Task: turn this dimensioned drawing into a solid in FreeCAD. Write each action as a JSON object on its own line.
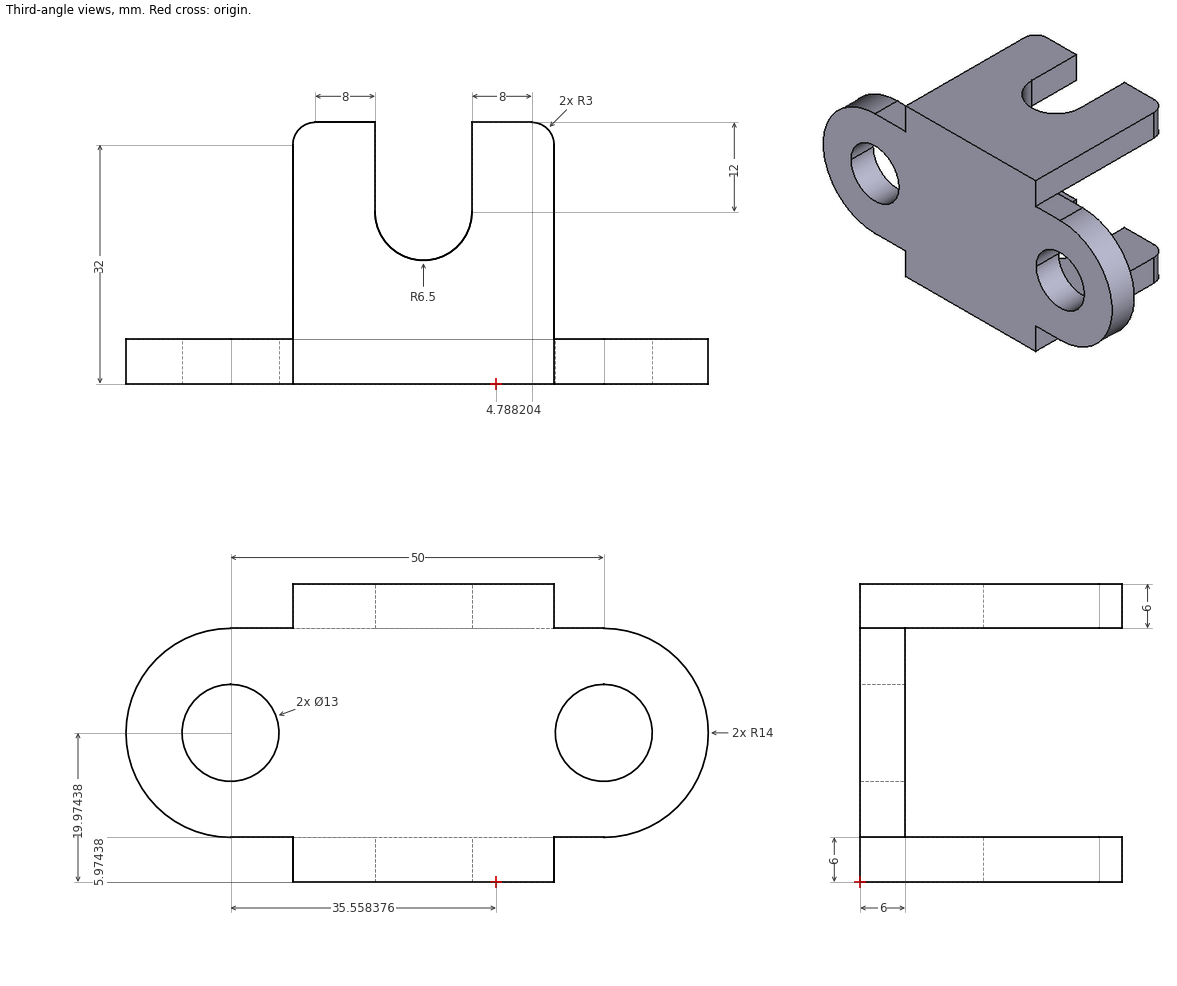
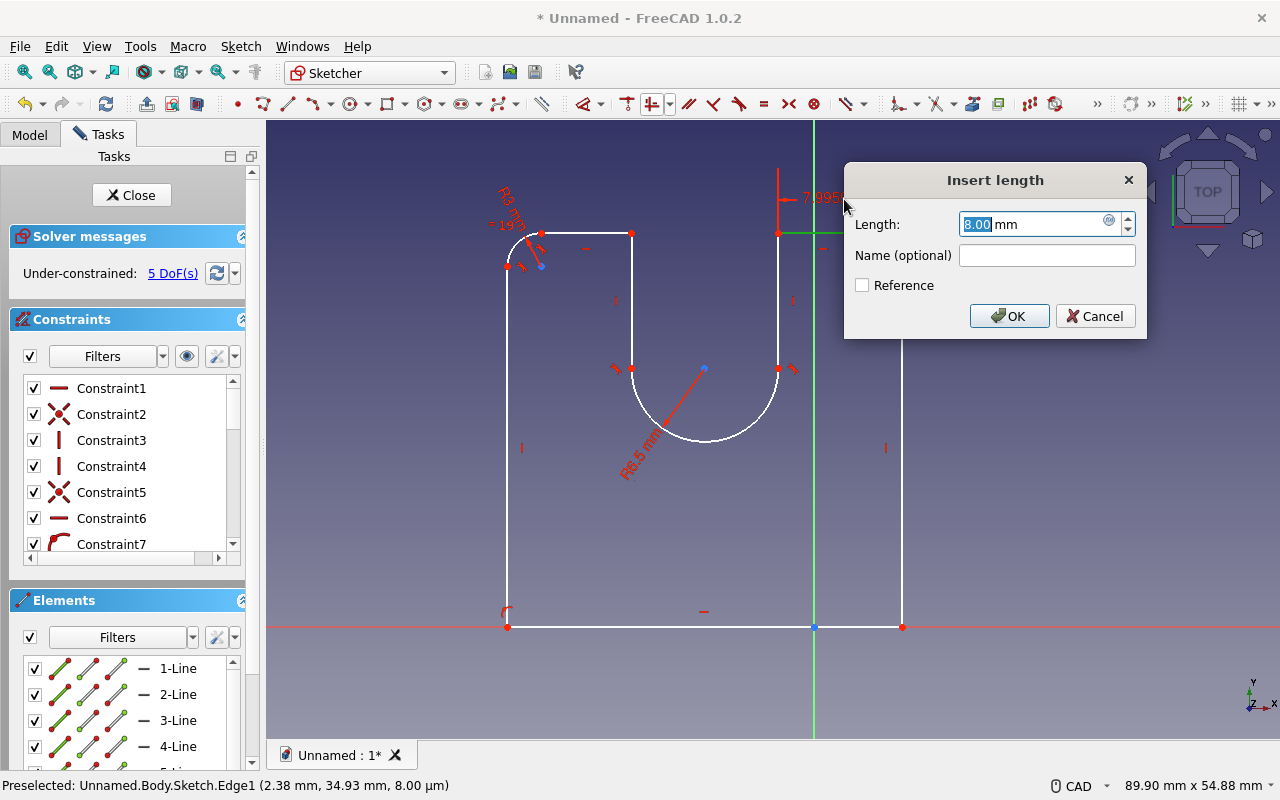
{"action": "type", "text": "8"}
{"action": "key", "text": "Return"}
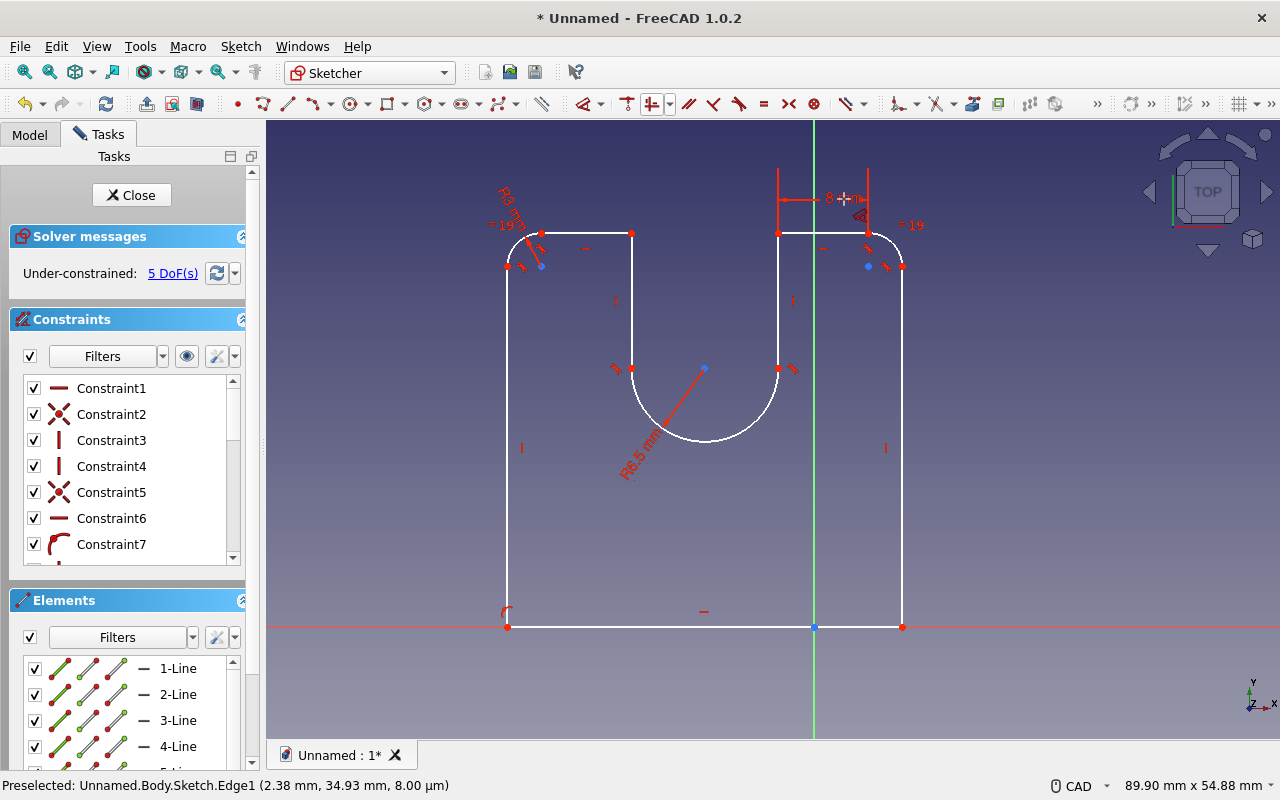
{"action": "left_click", "coordinate": [604, 233]}
{"action": "left_click", "coordinate": [586, 199]}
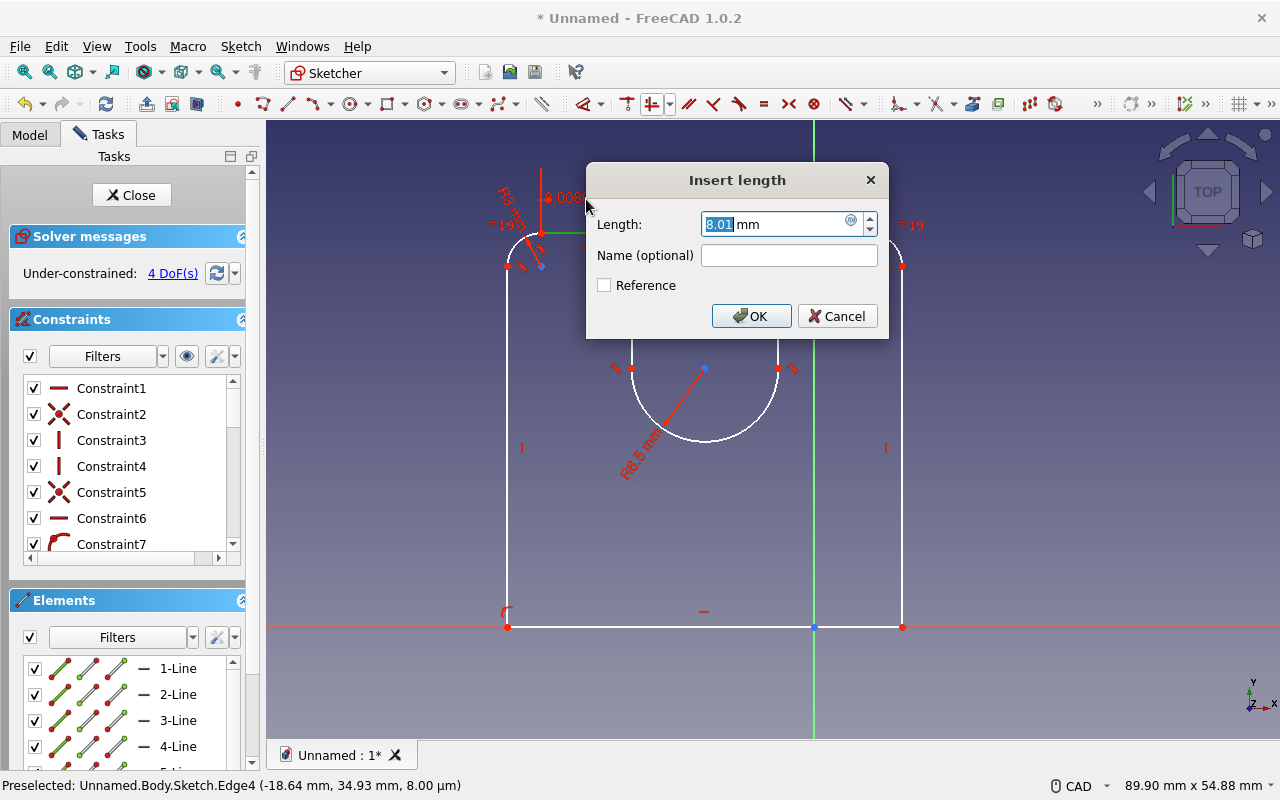
{"action": "type", "text": "8"}
{"action": "key", "text": "Return"}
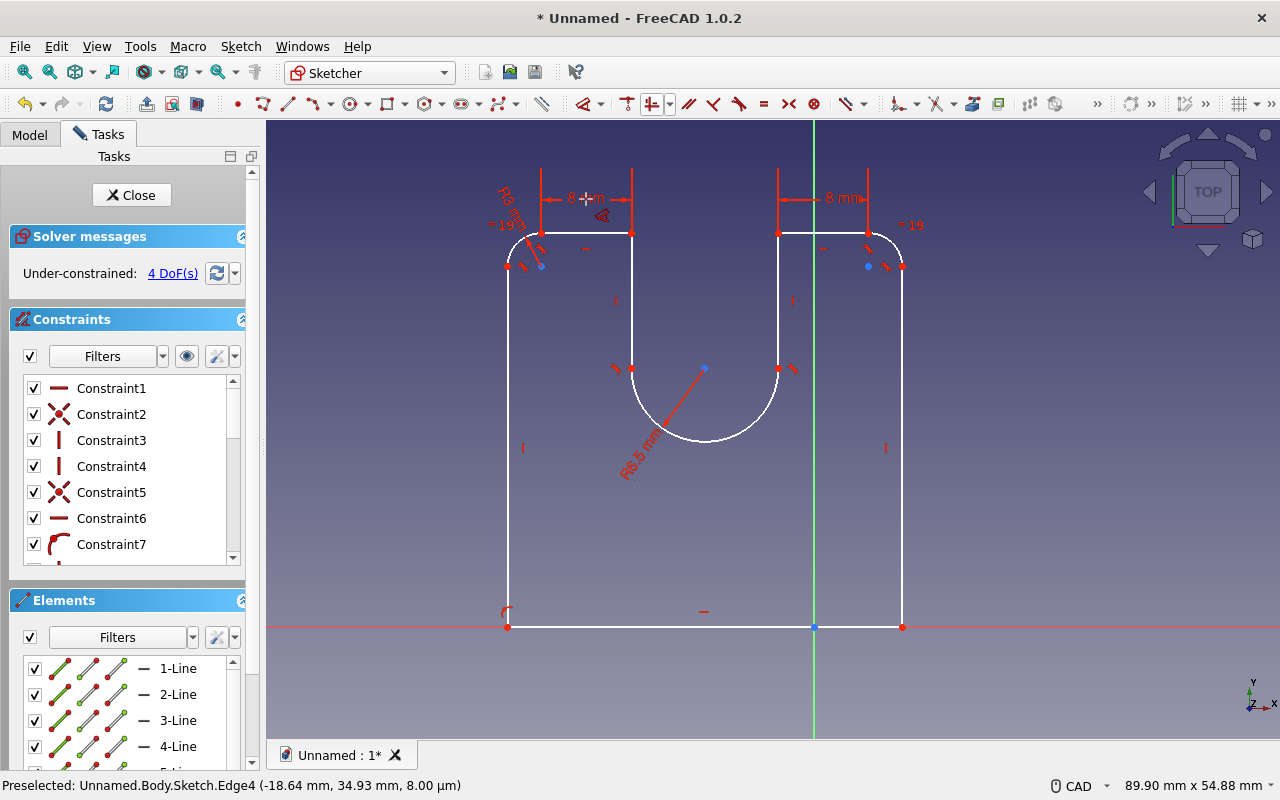
{"action": "left_click", "coordinate": [778, 274]}
{"action": "left_click", "coordinate": [744, 301]}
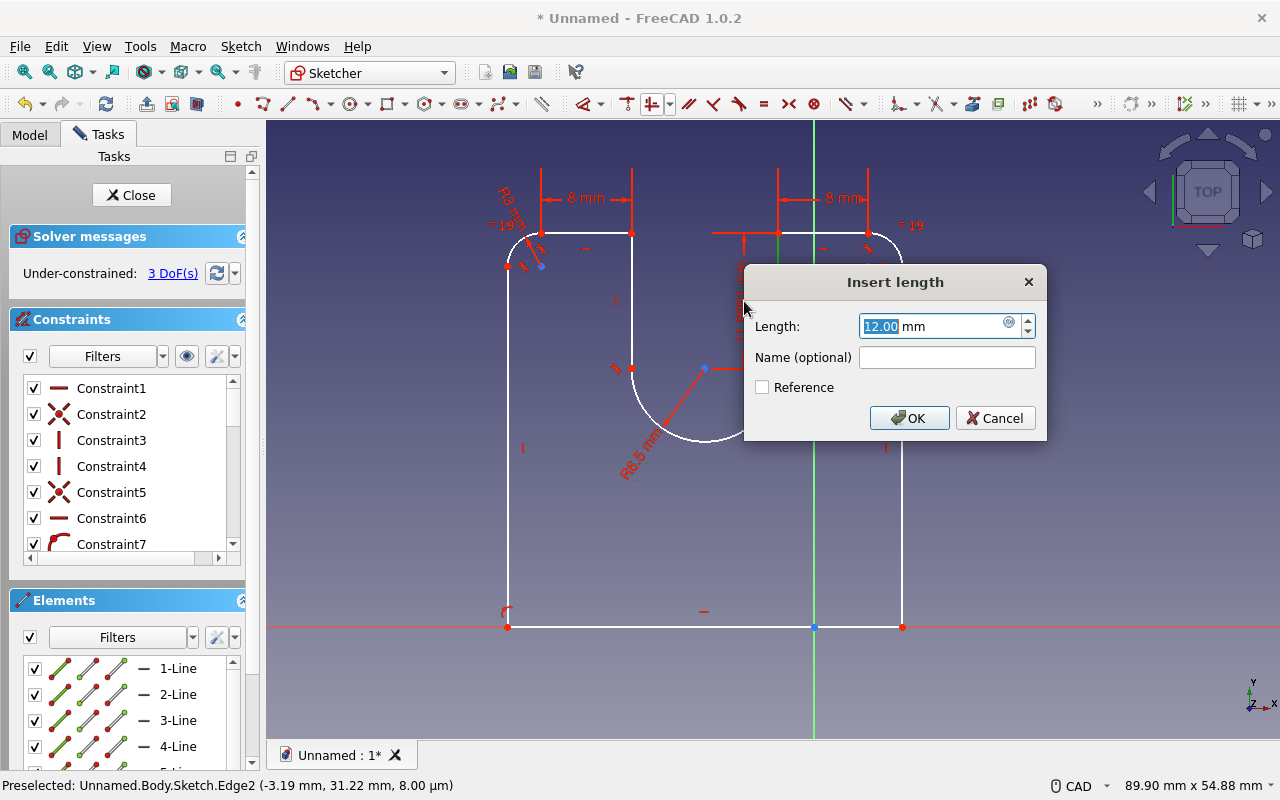
{"action": "type", "text": "12"}
{"action": "key", "text": "Return"}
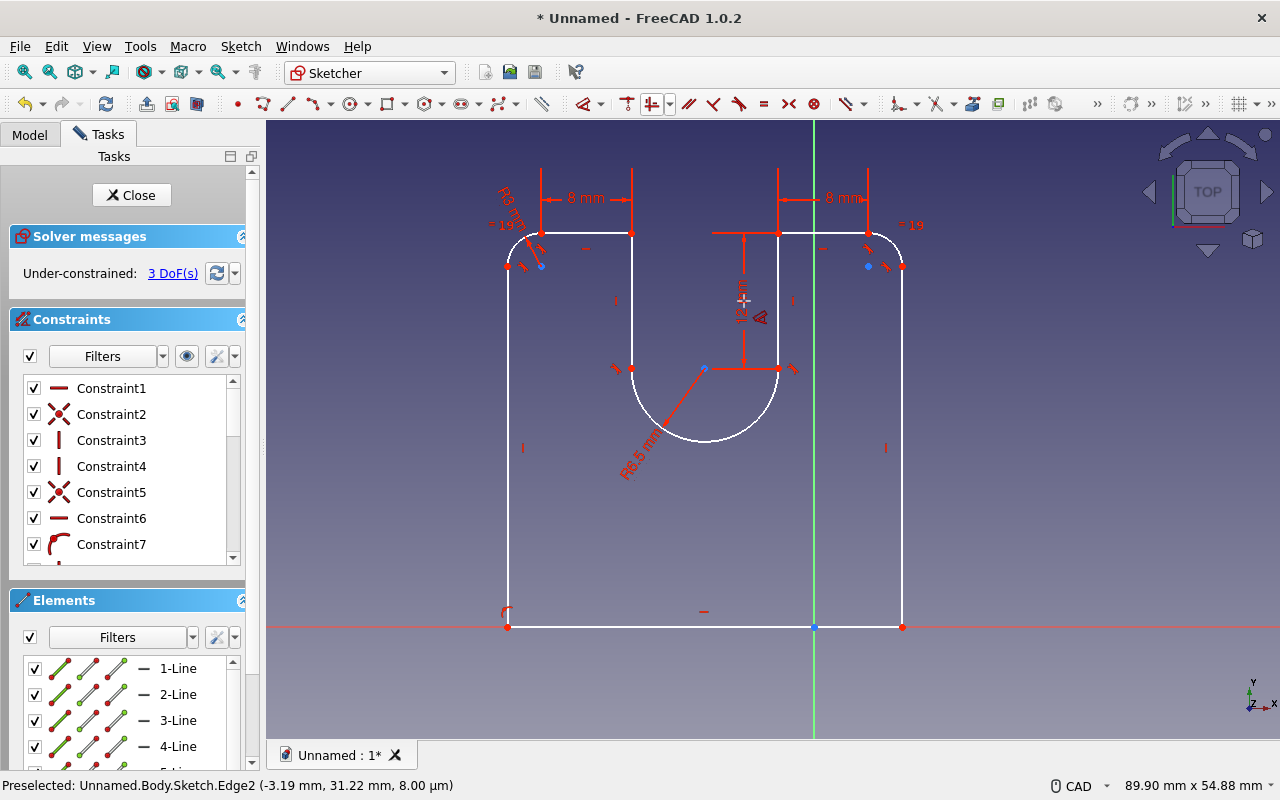
{"action": "left_click", "coordinate": [632, 328]}
{"action": "left_click", "coordinate": [598, 301]}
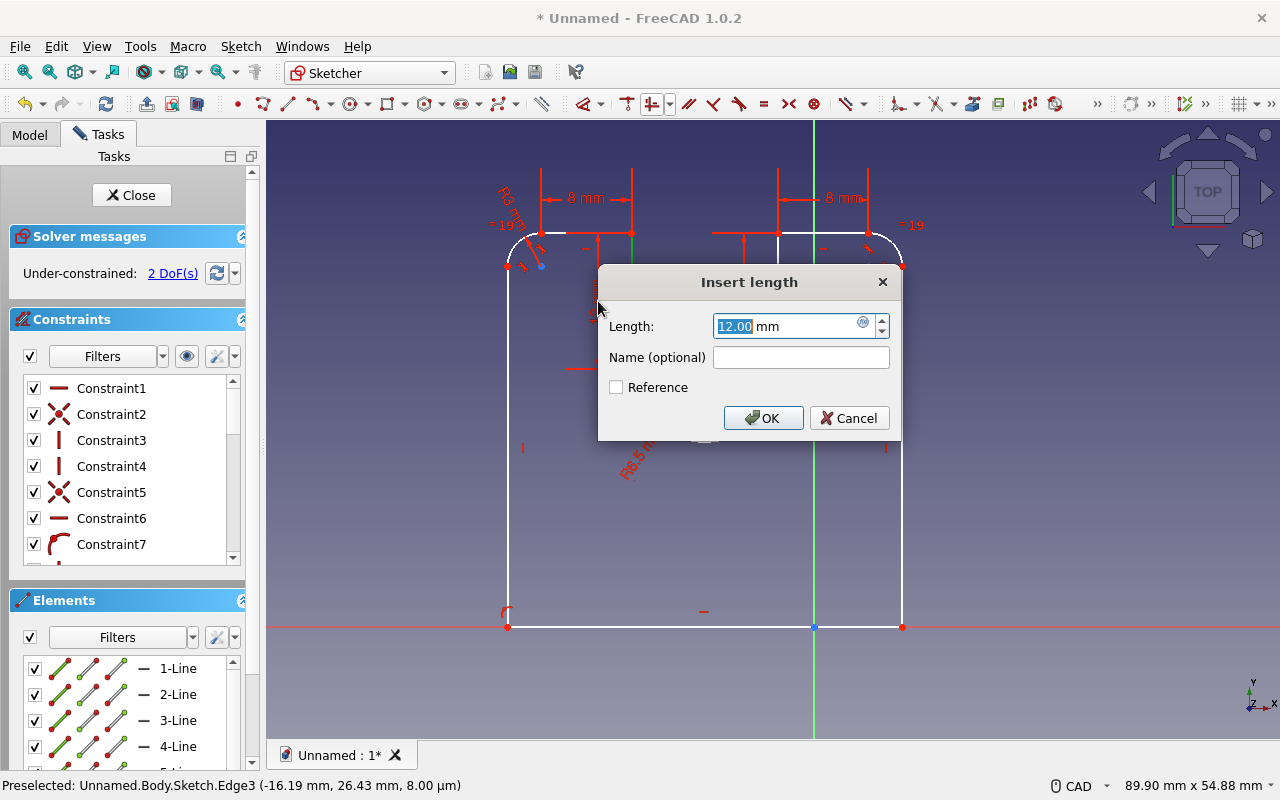
{"action": "type", "text": "12"}
{"action": "key", "text": "Return"}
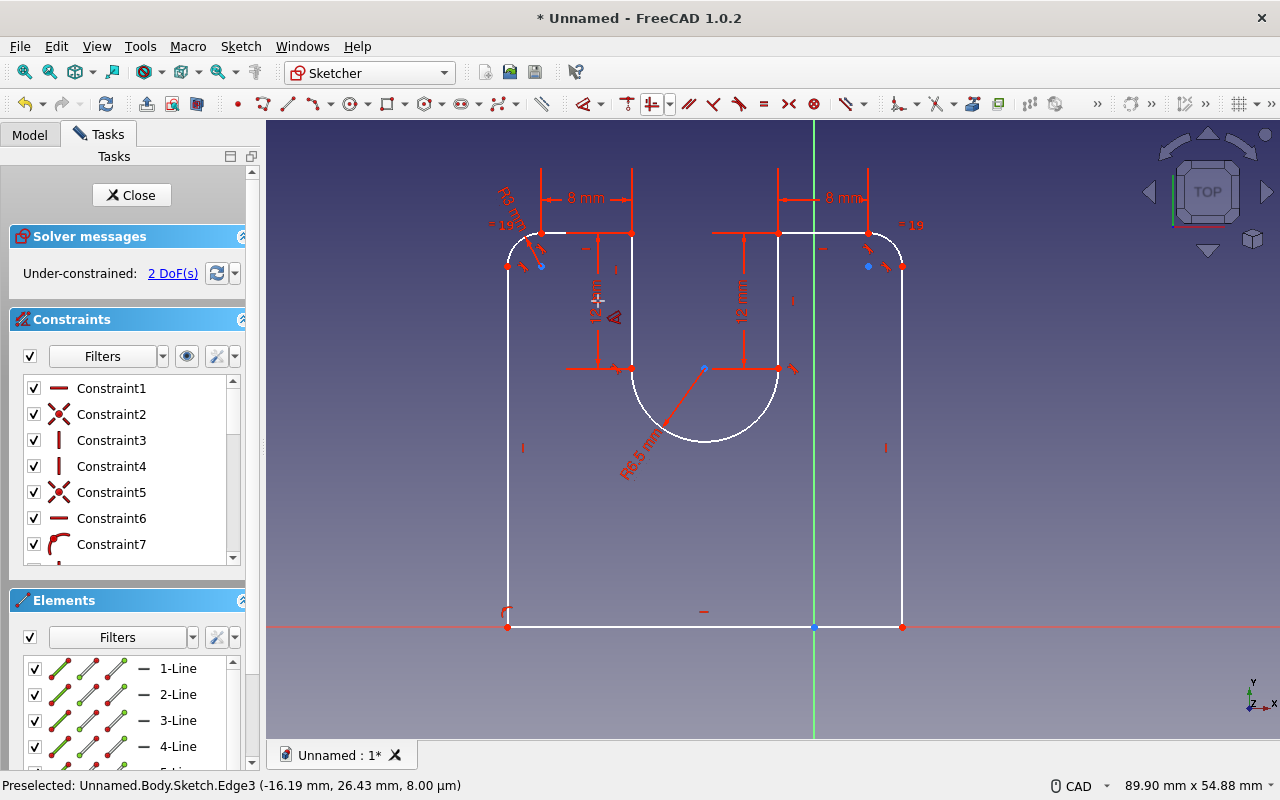
{"action": "left_click", "coordinate": [508, 375]}
{"action": "left_click", "coordinate": [474, 447]}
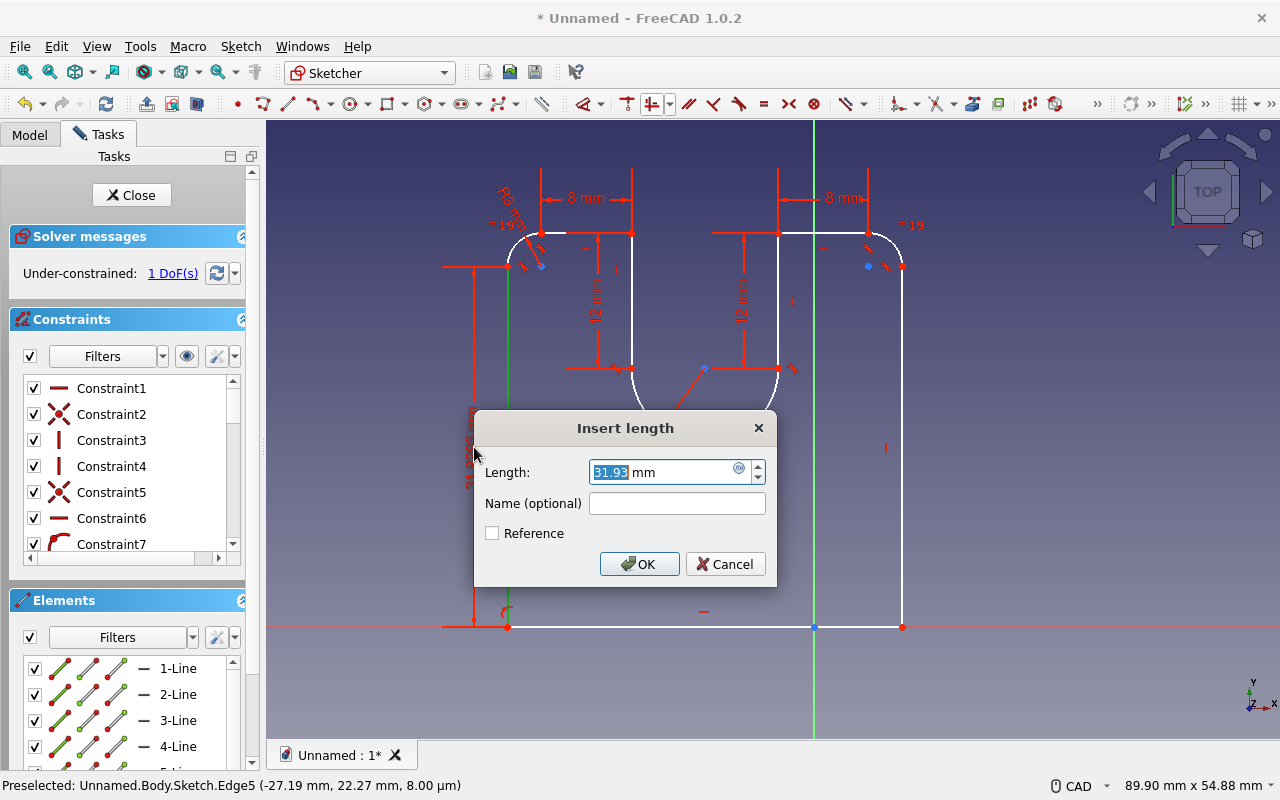
{"action": "type", "text": "32"}
{"action": "key", "text": "Return"}